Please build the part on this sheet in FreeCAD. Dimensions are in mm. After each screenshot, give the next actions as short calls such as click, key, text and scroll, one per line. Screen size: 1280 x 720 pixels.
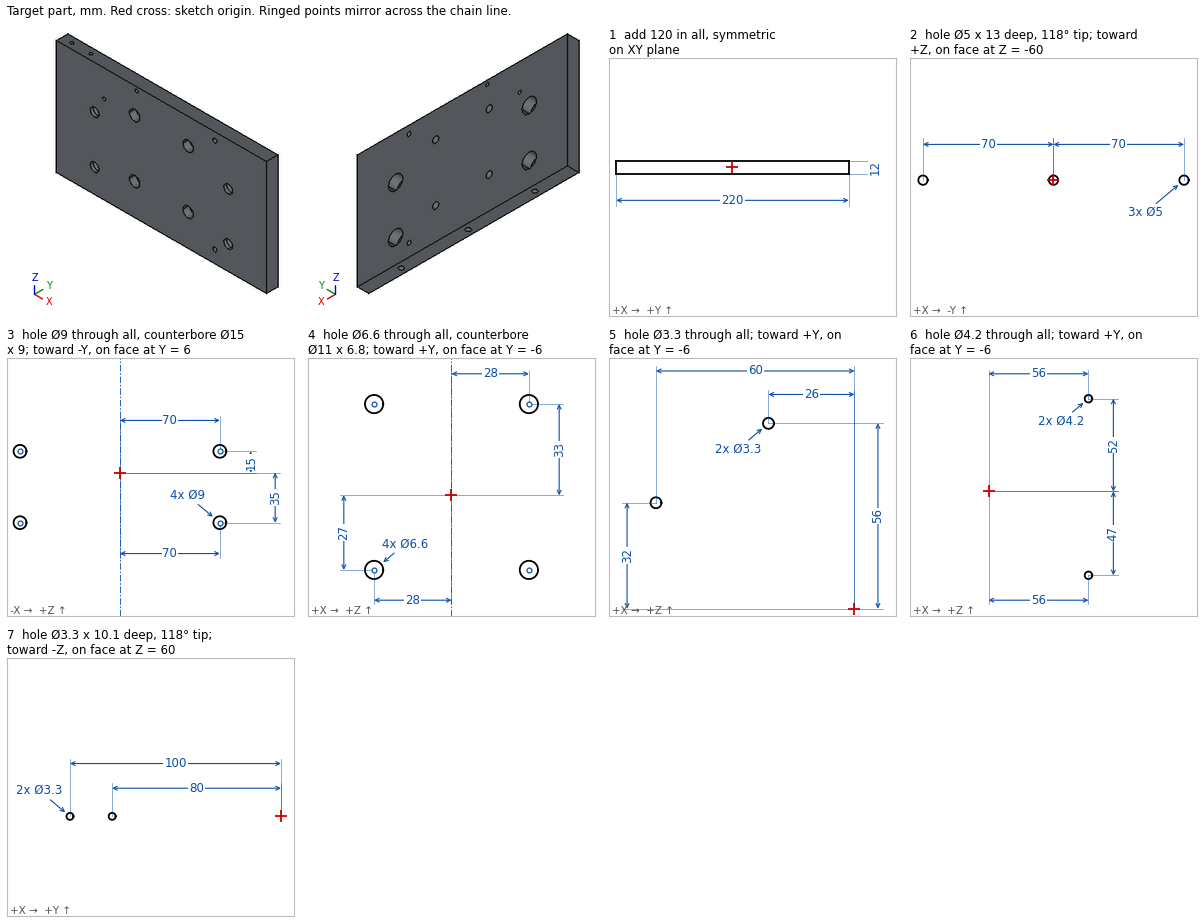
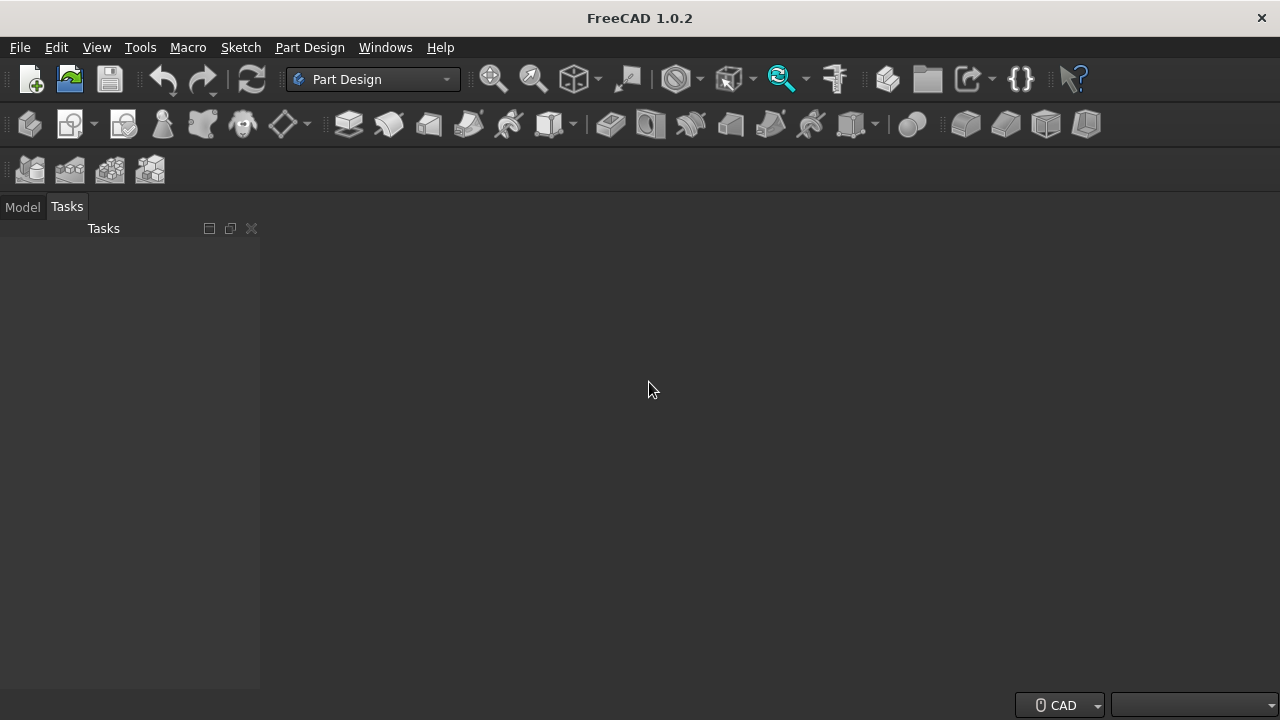
click(30, 80)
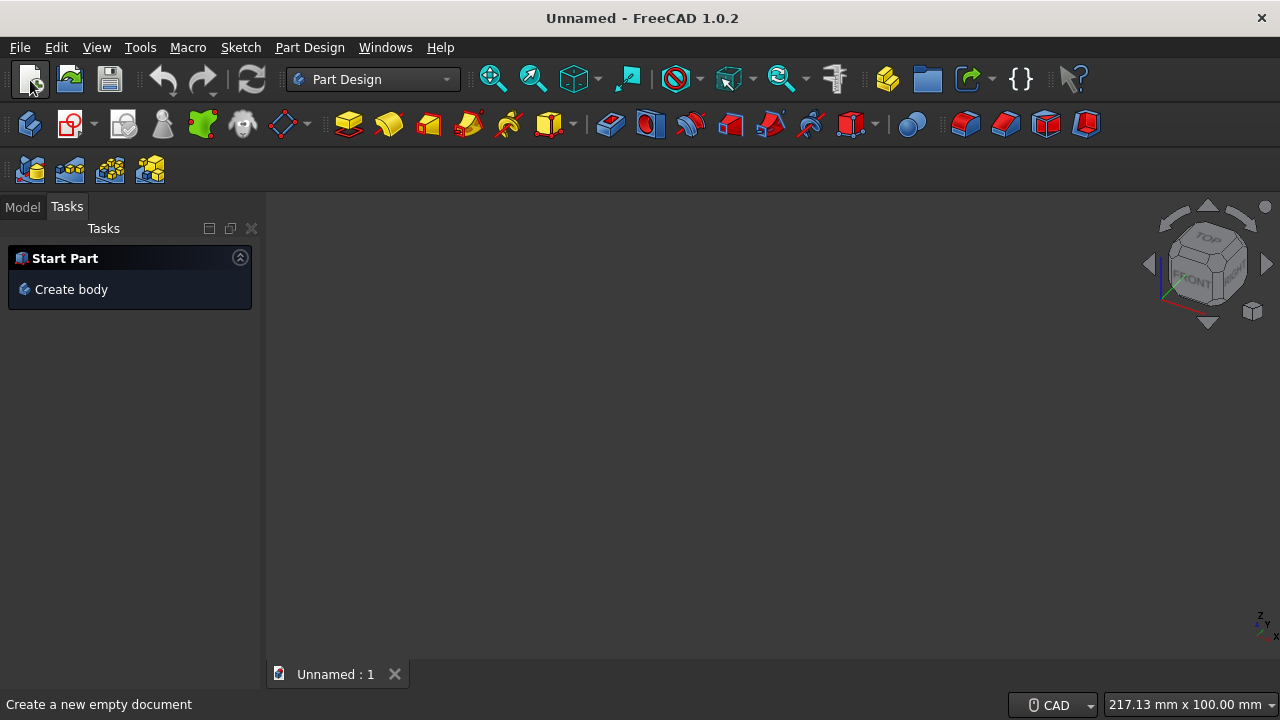
click(70, 124)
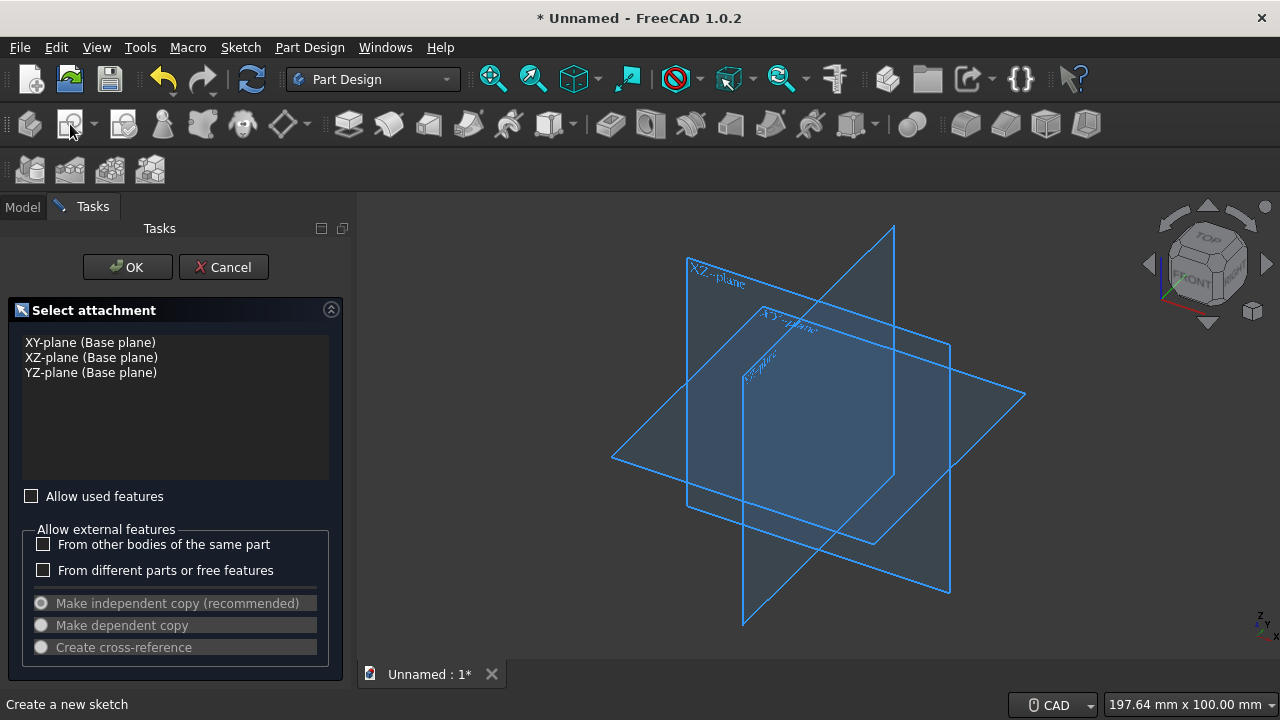
click(82, 342)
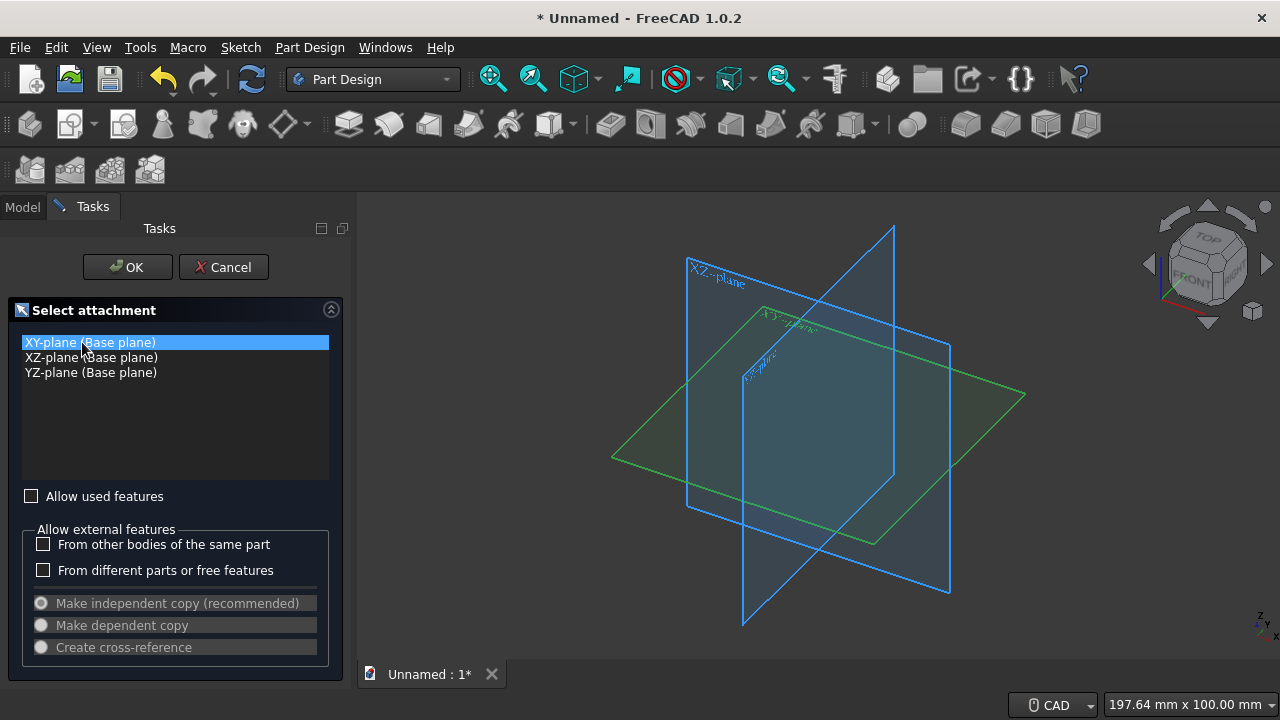
click(128, 267)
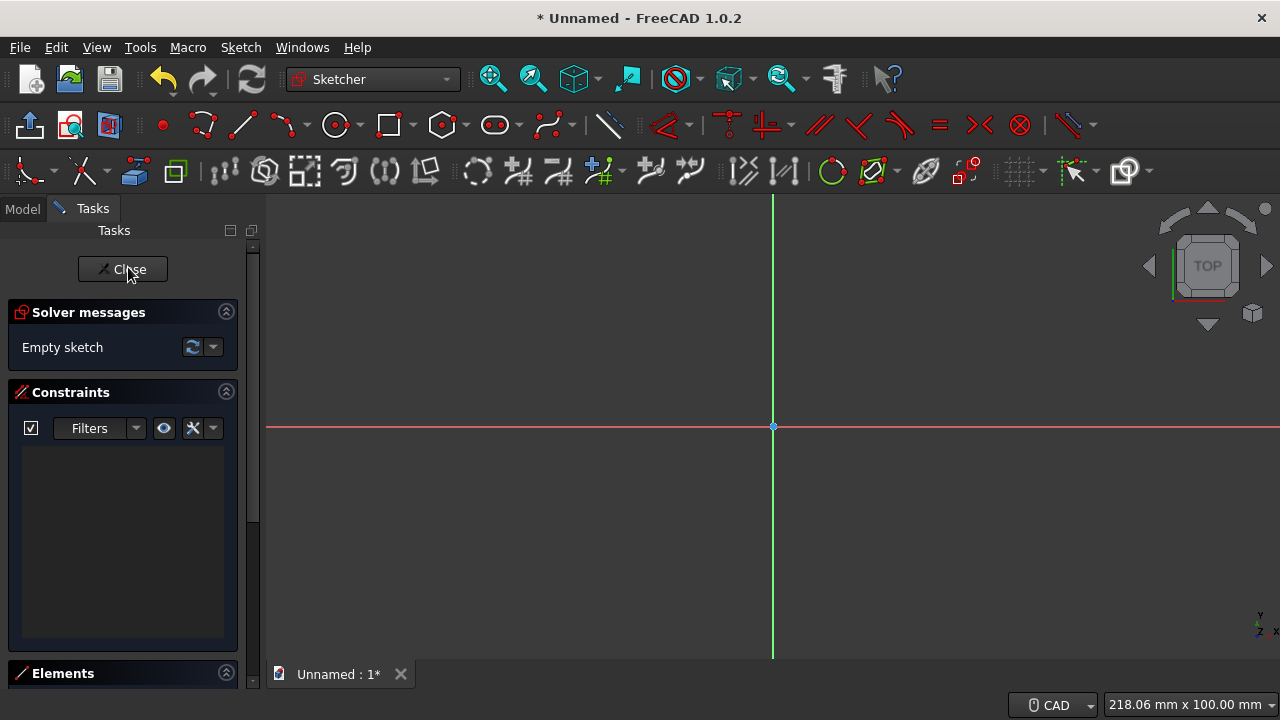
scroll(621, 426, down, 3)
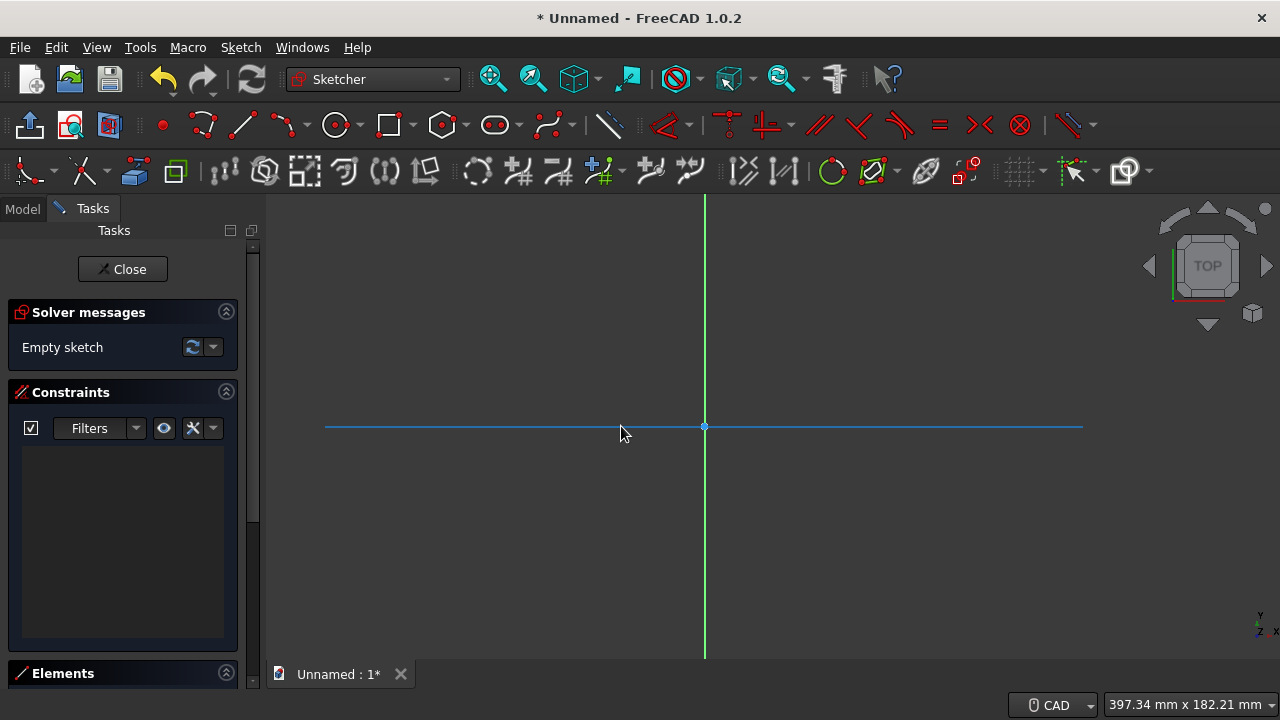
key(g)
key(v)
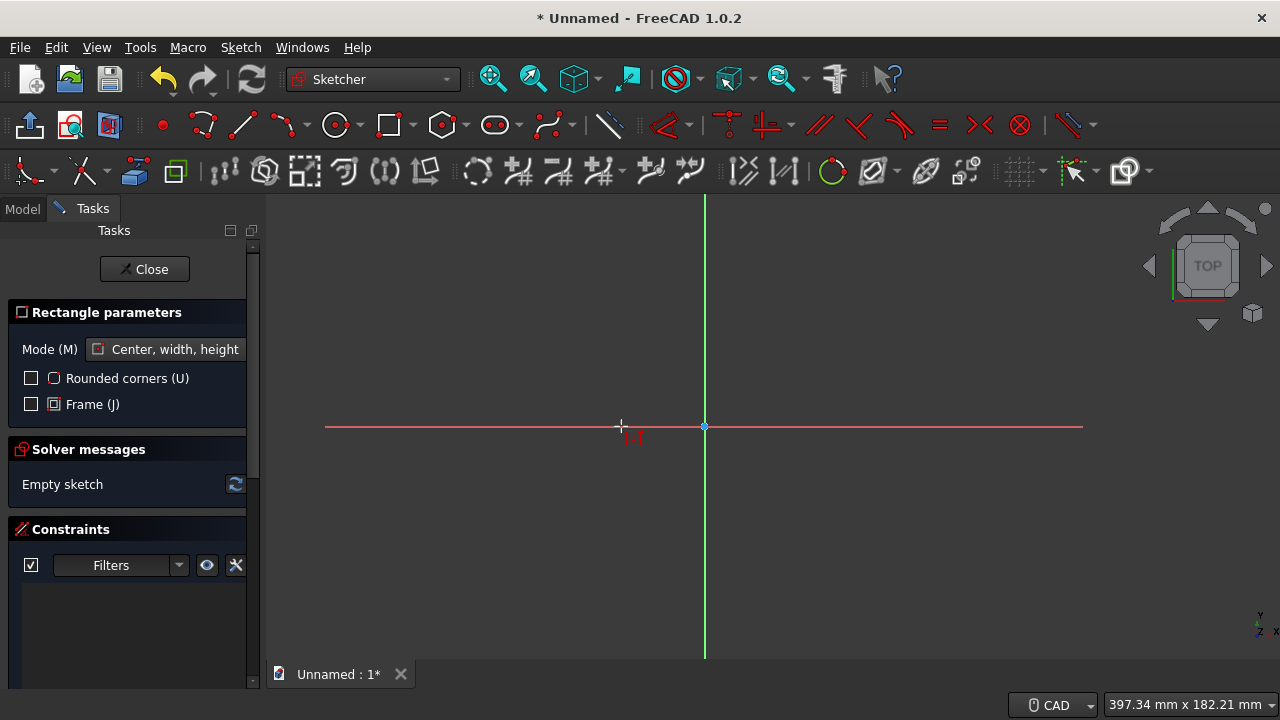
click(705, 426)
move(985, 411)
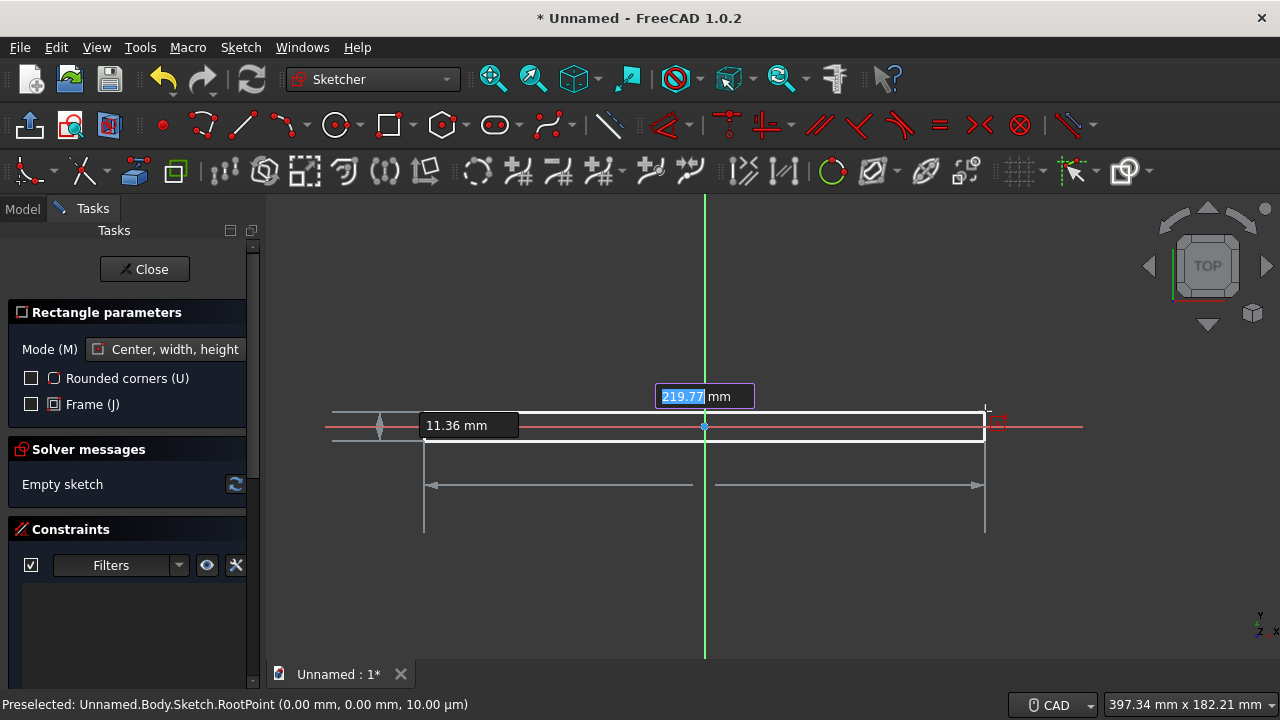
text(220)
key(Tab)
text(12)
key(Return)
key(Escape)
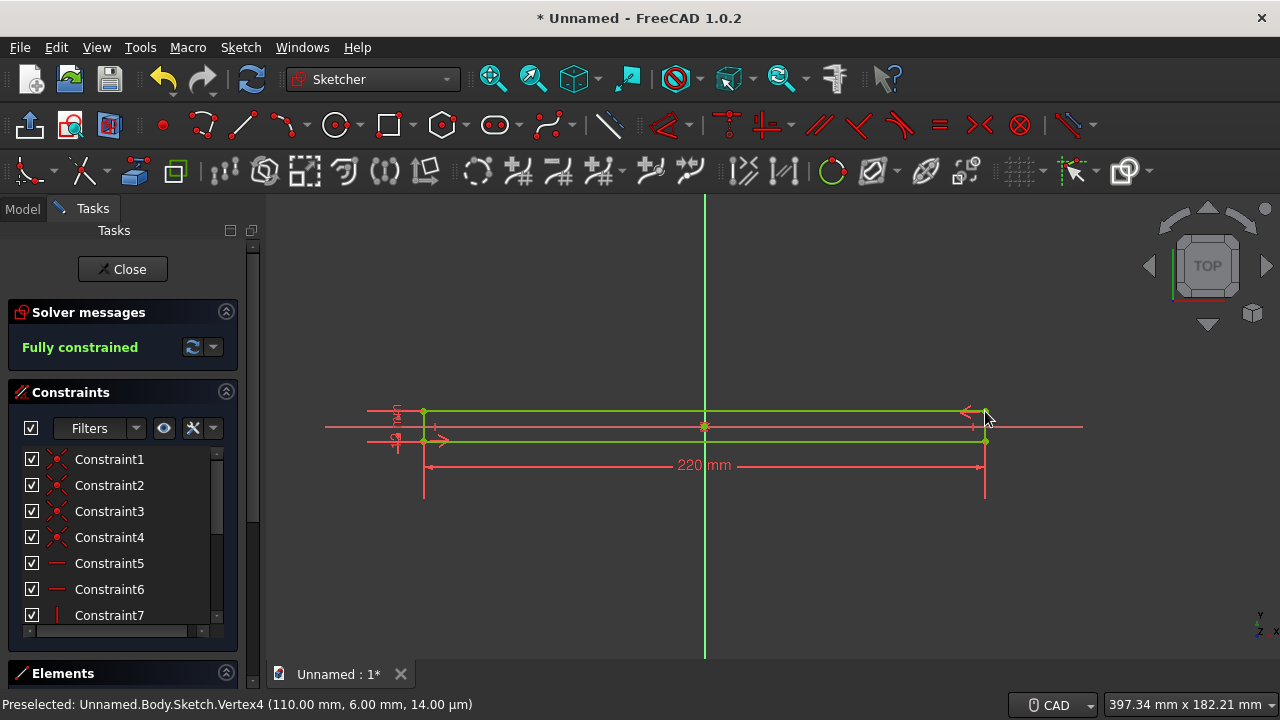
click(123, 269)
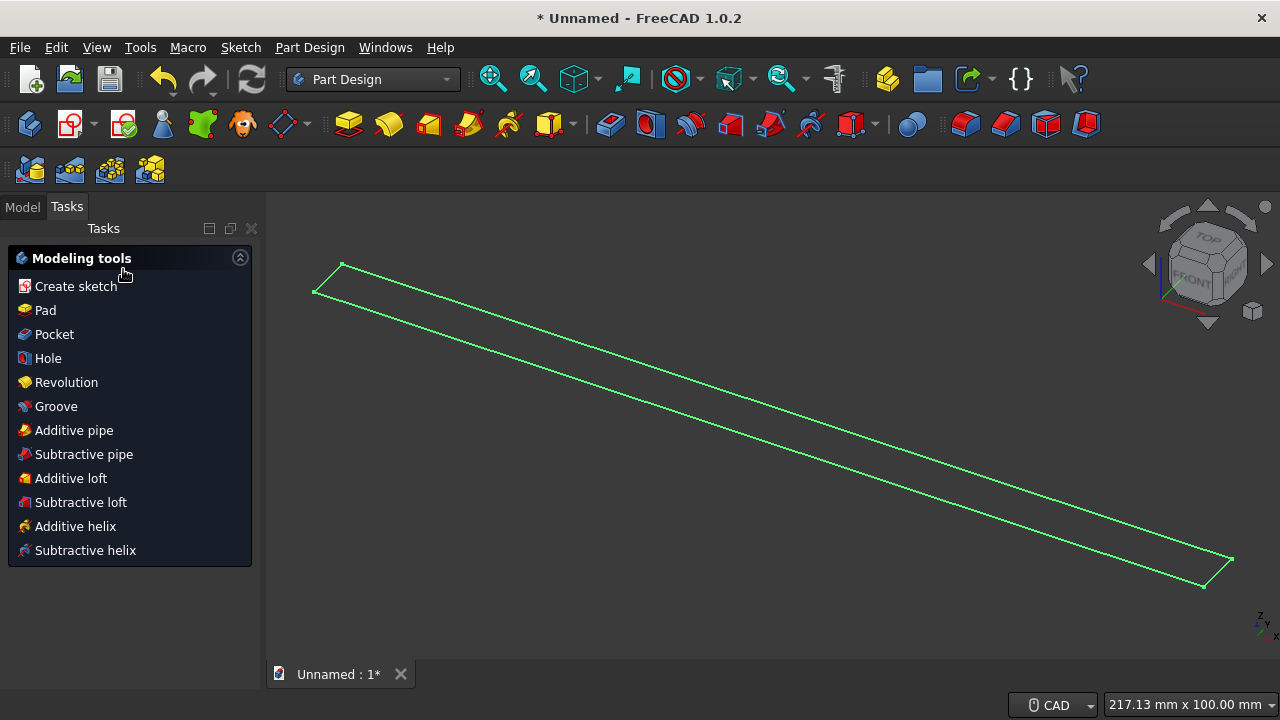
click(350, 124)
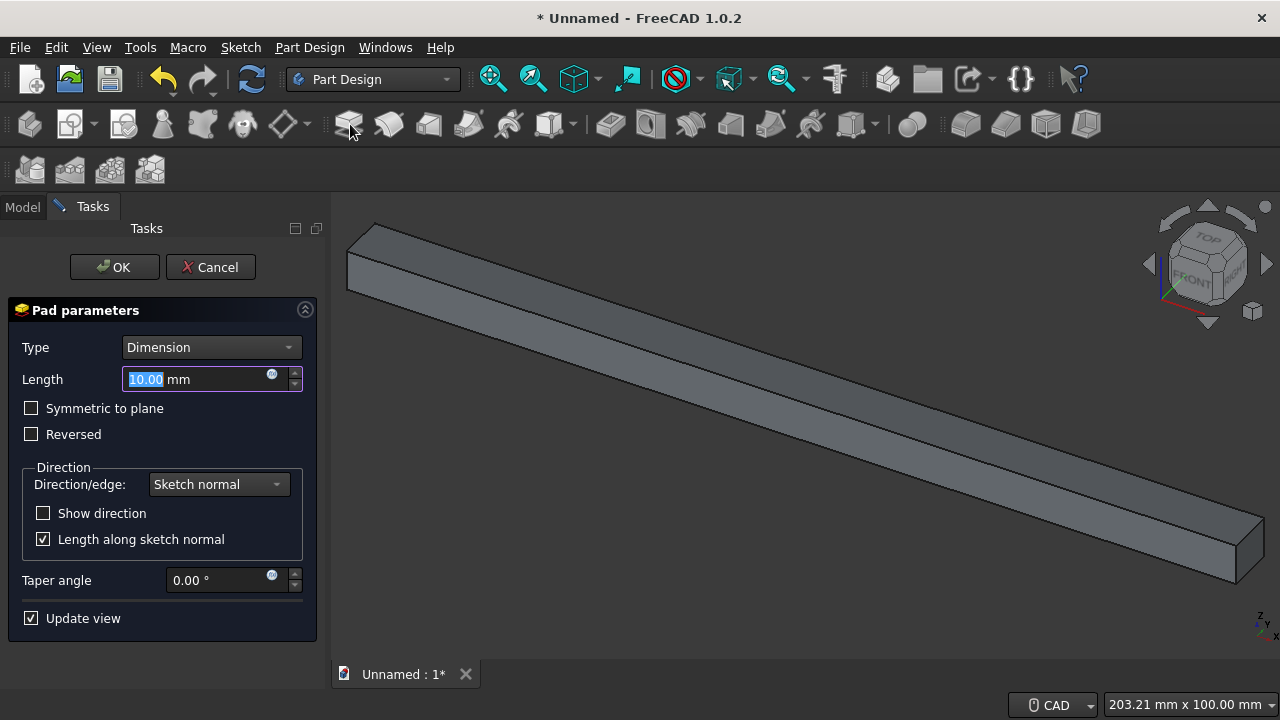
text(120)
key(Tab)